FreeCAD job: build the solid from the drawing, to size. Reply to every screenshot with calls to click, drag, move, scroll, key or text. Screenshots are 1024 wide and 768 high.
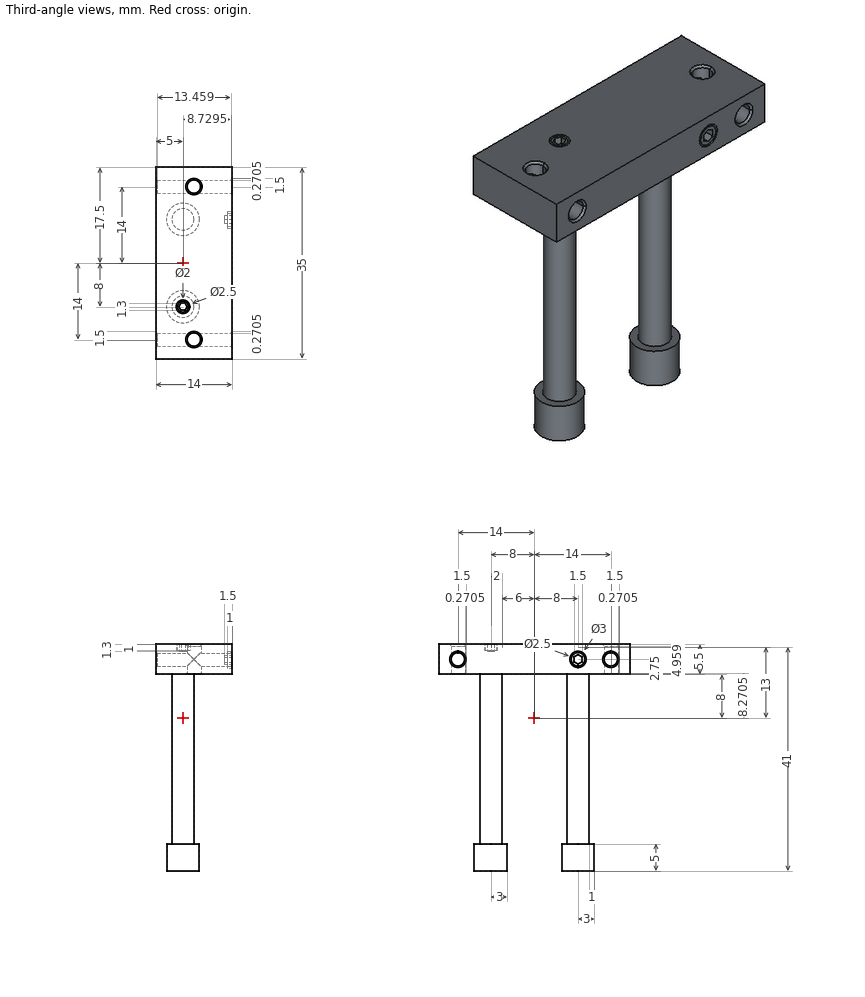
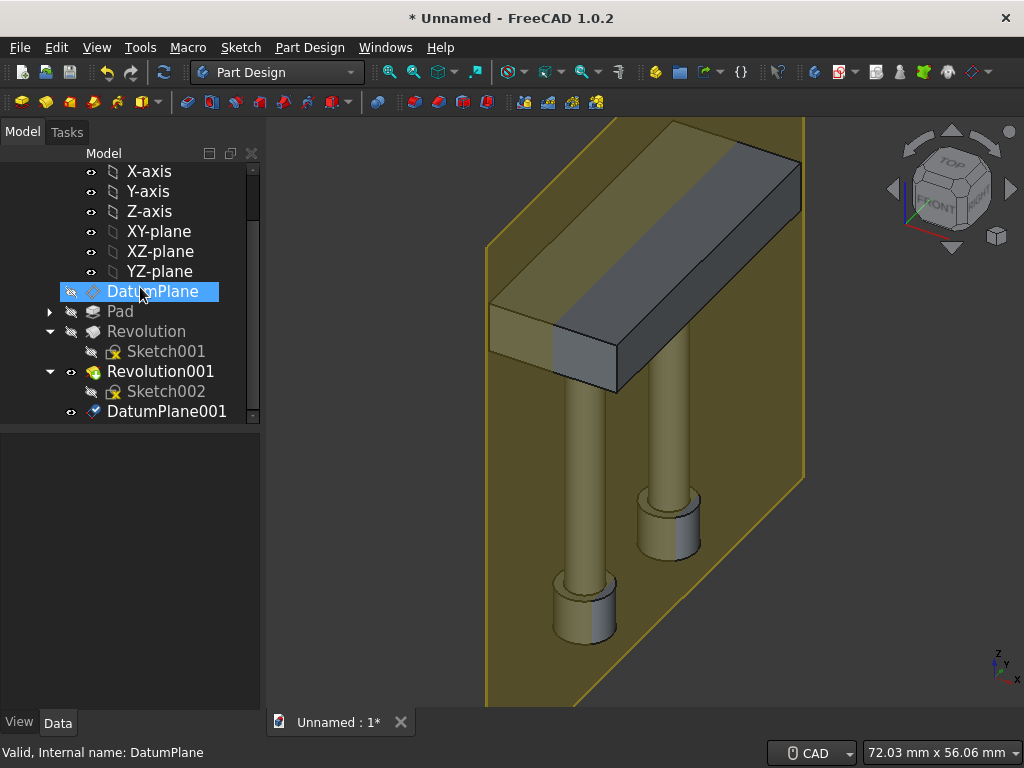
click(116, 412)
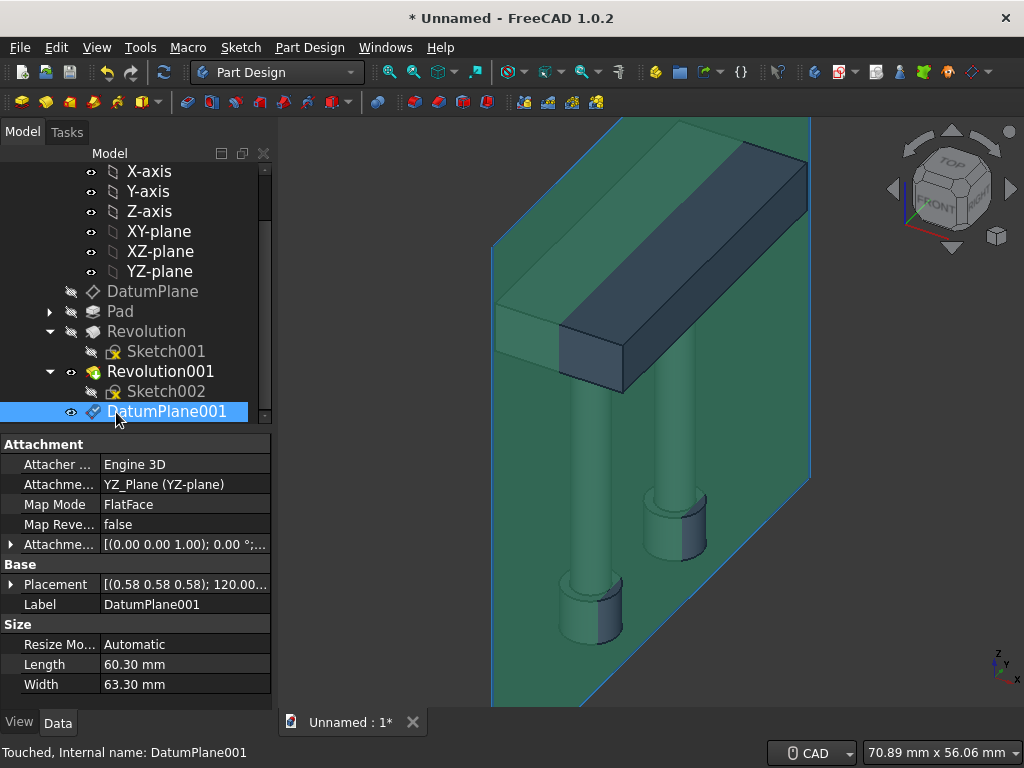
click(840, 72)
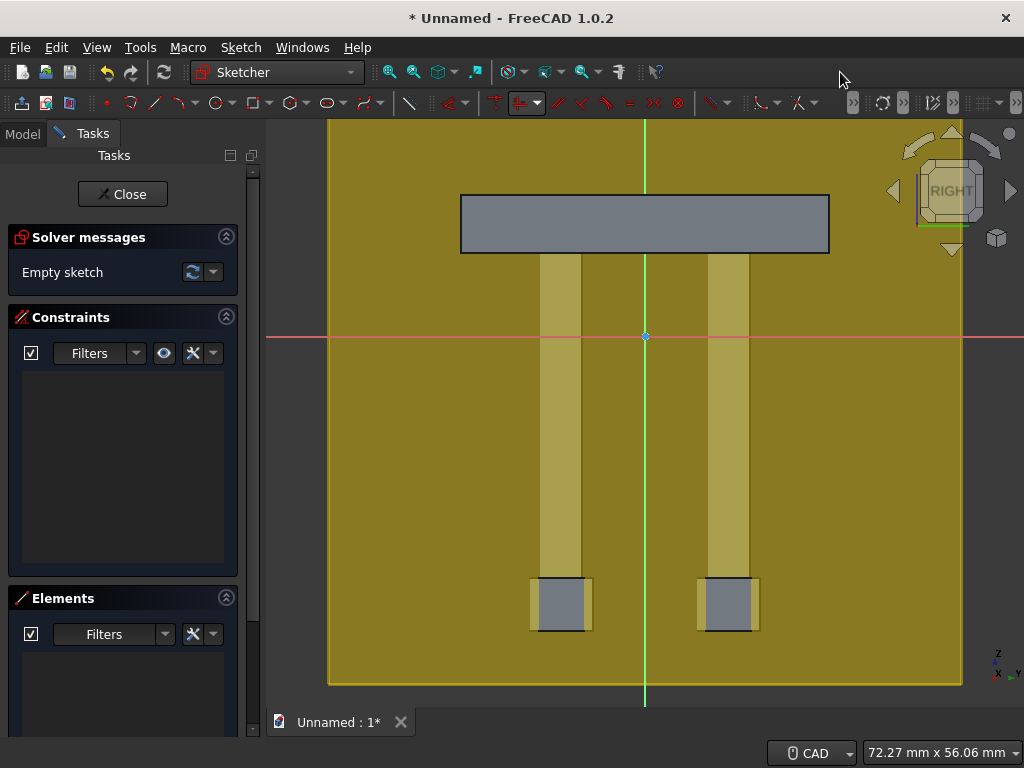
click(70, 104)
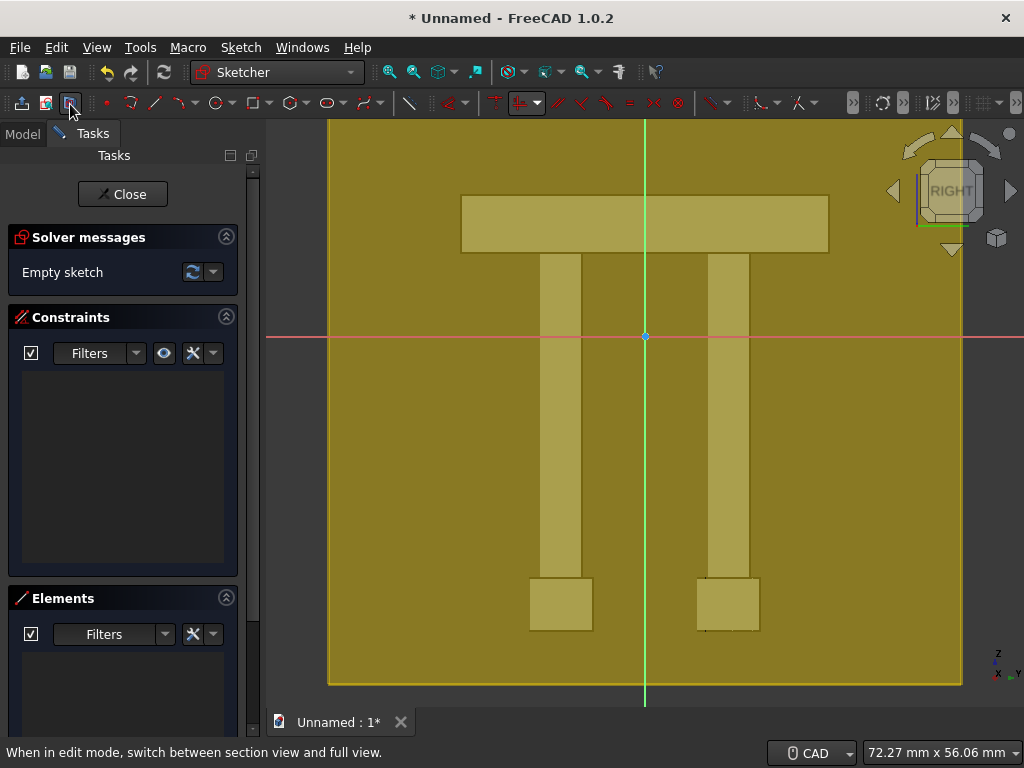
scroll(848, 147, up, 4)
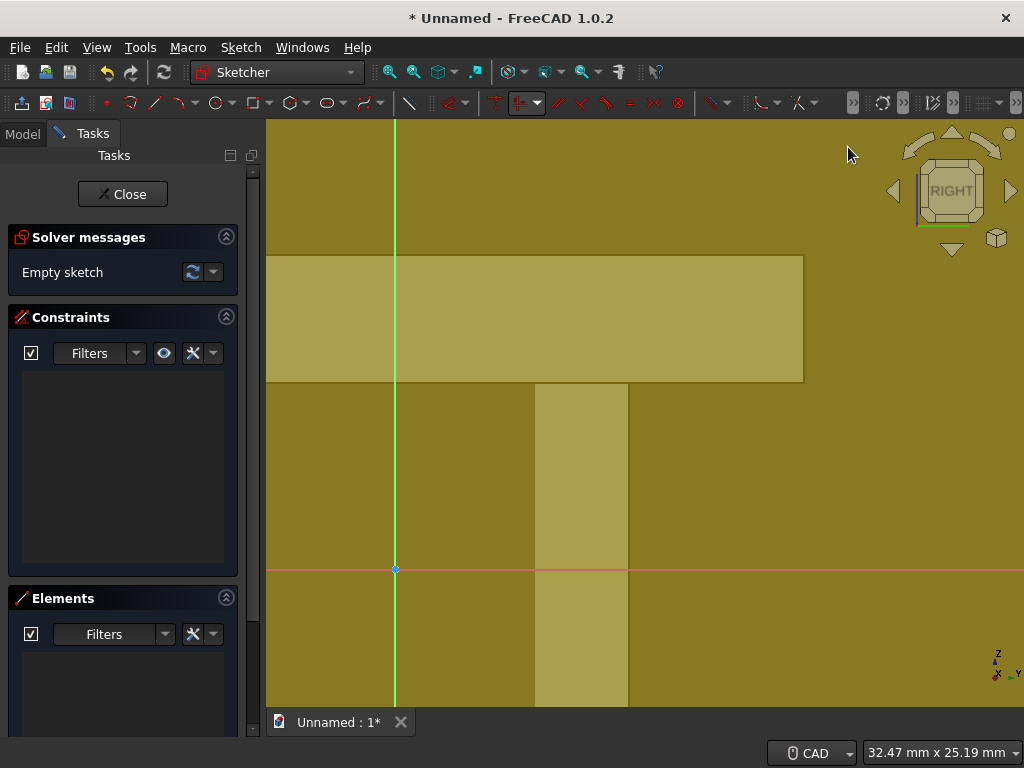
click(132, 104)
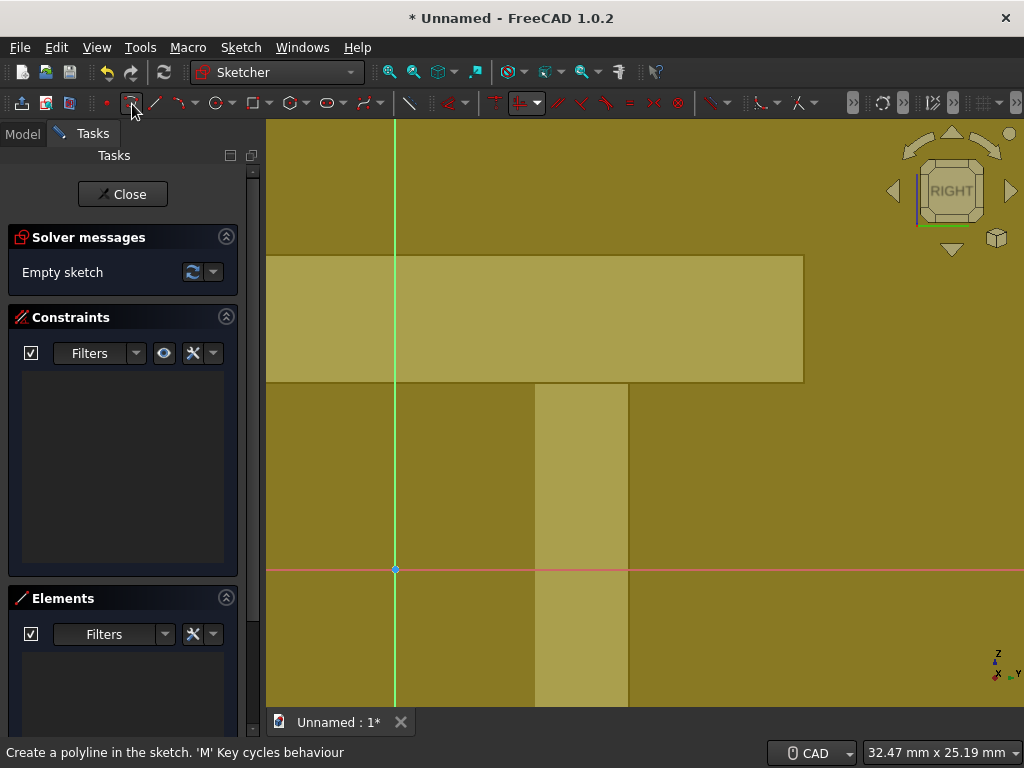
click(722, 383)
click(757, 383)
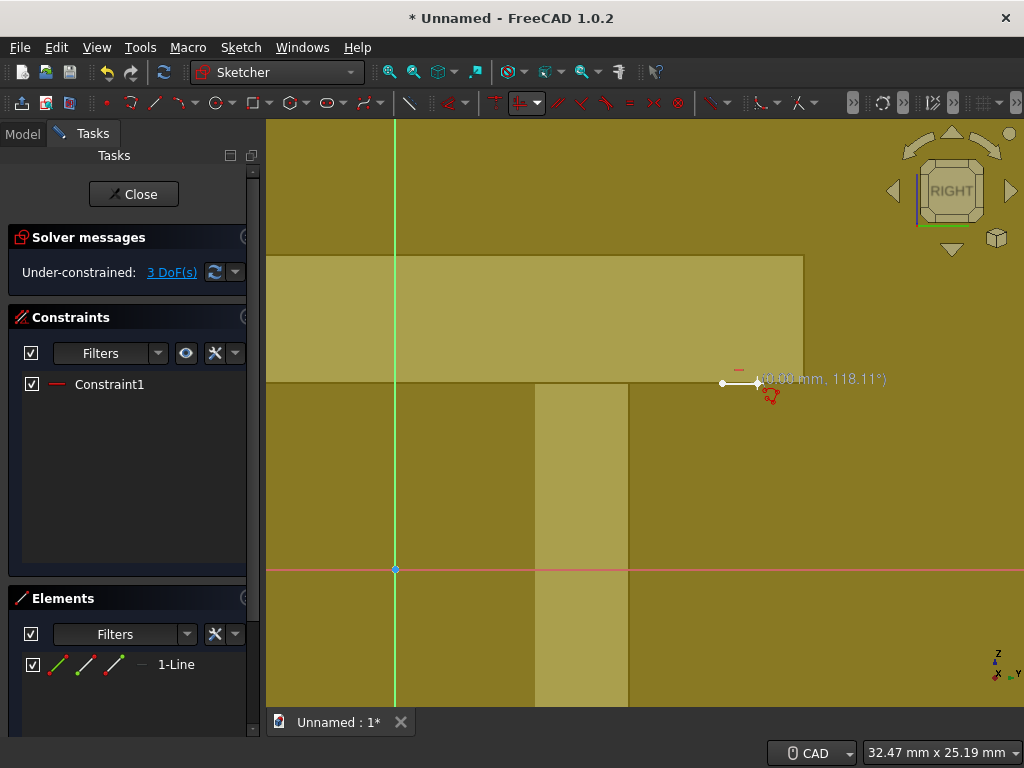
scroll(751, 377, up, 5)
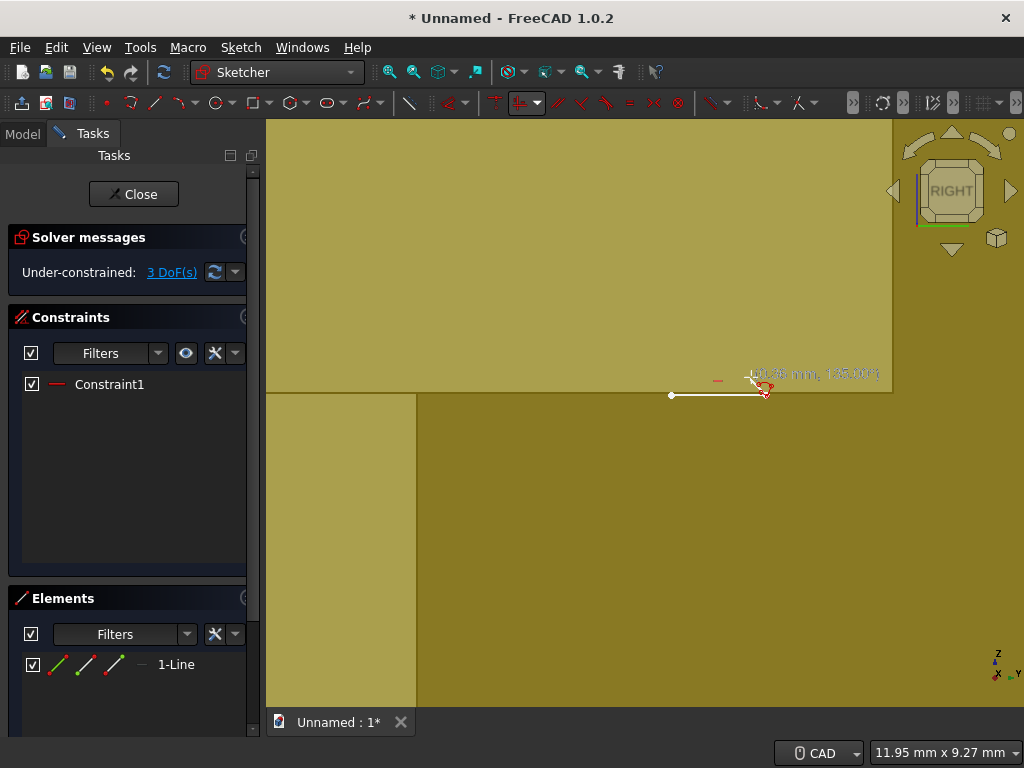
click(749, 375)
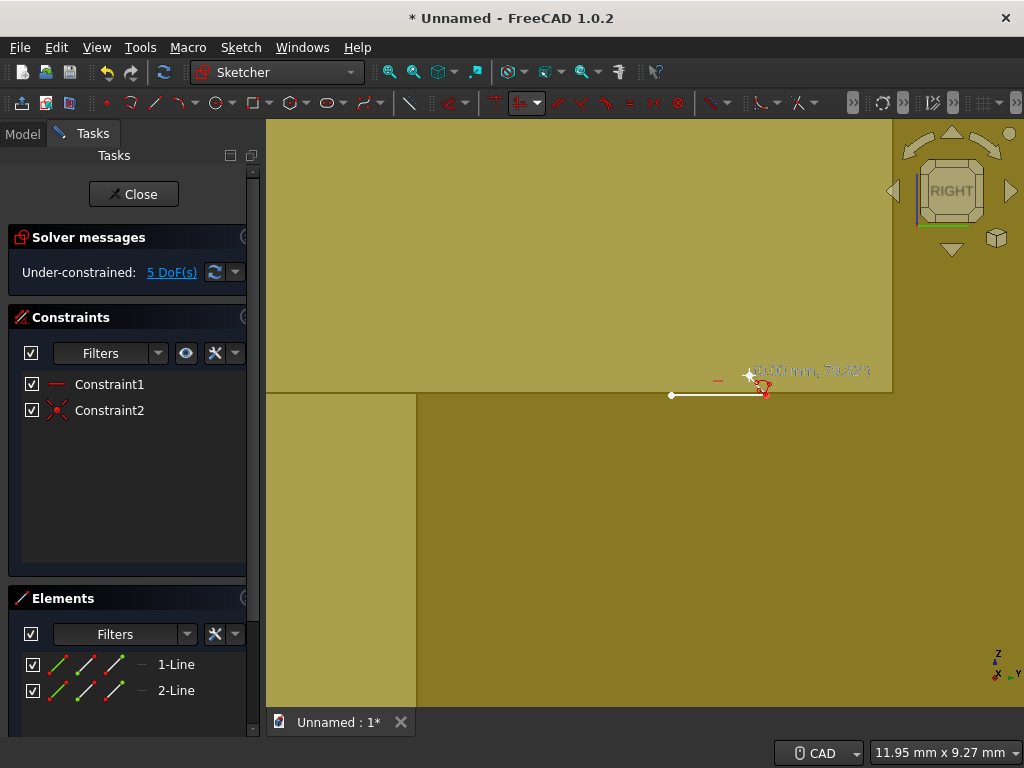
scroll(752, 419, down, 5)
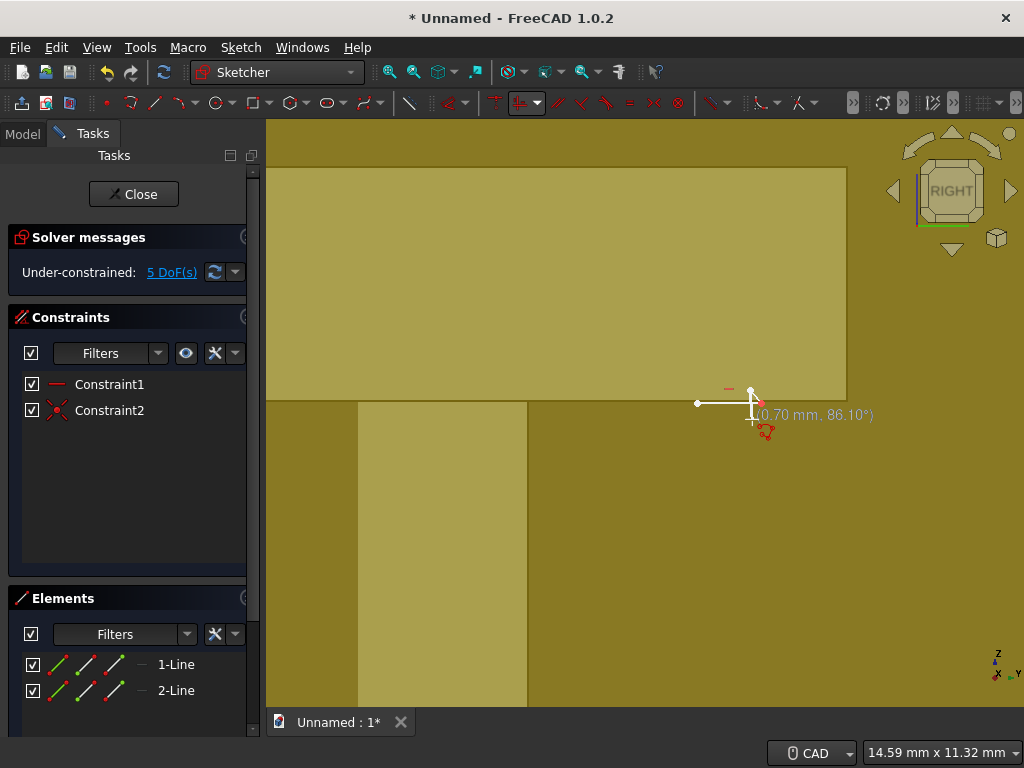
click(751, 288)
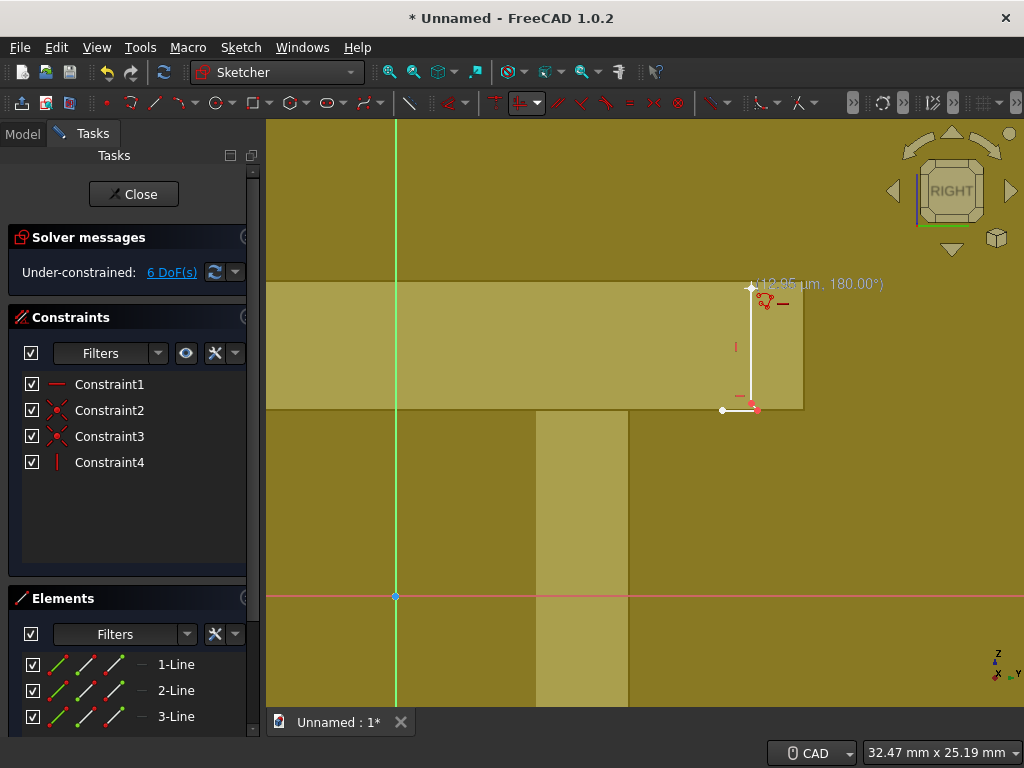
scroll(758, 281, up, 3)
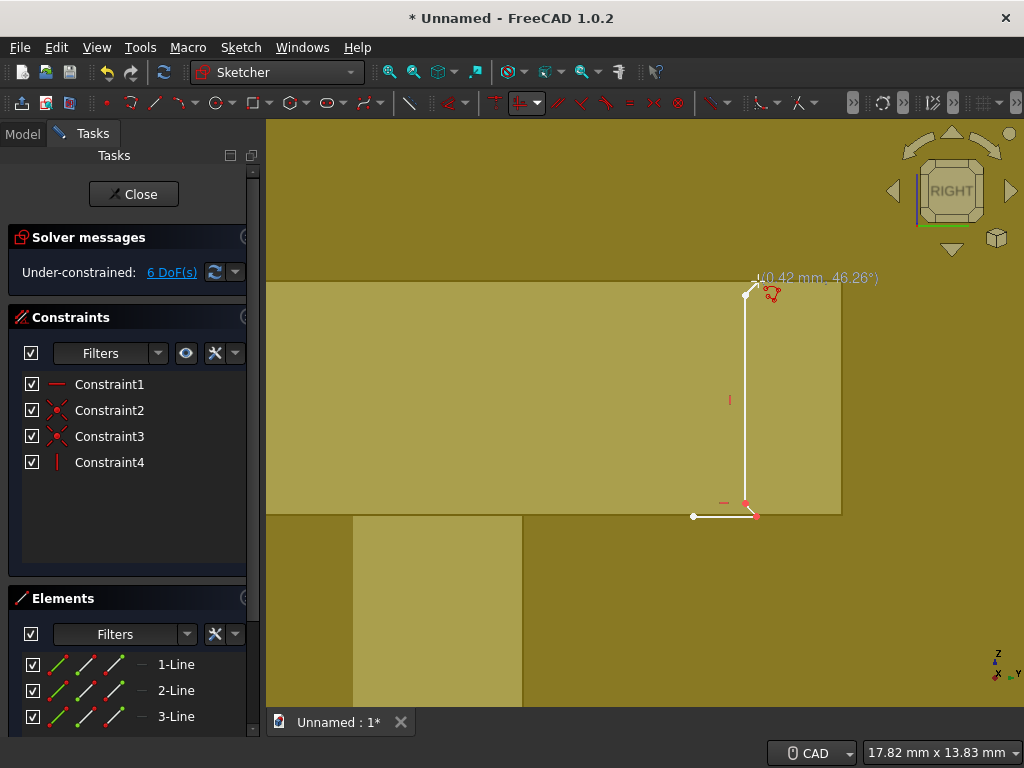
click(757, 281)
click(693, 281)
click(693, 517)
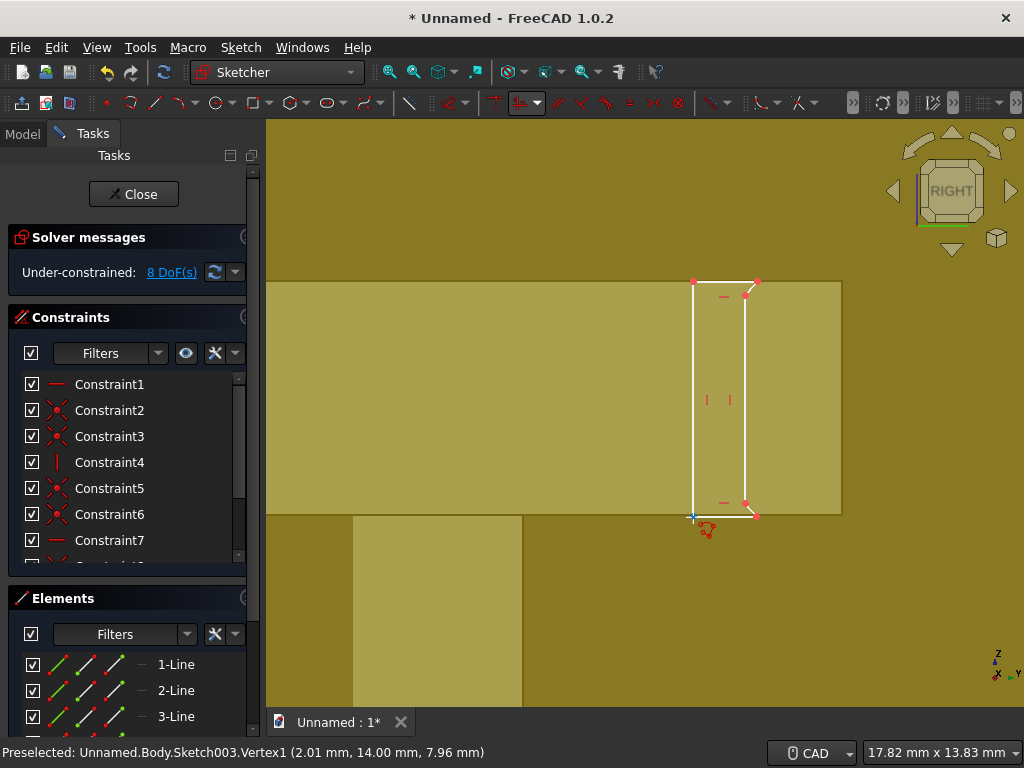
click(156, 104)